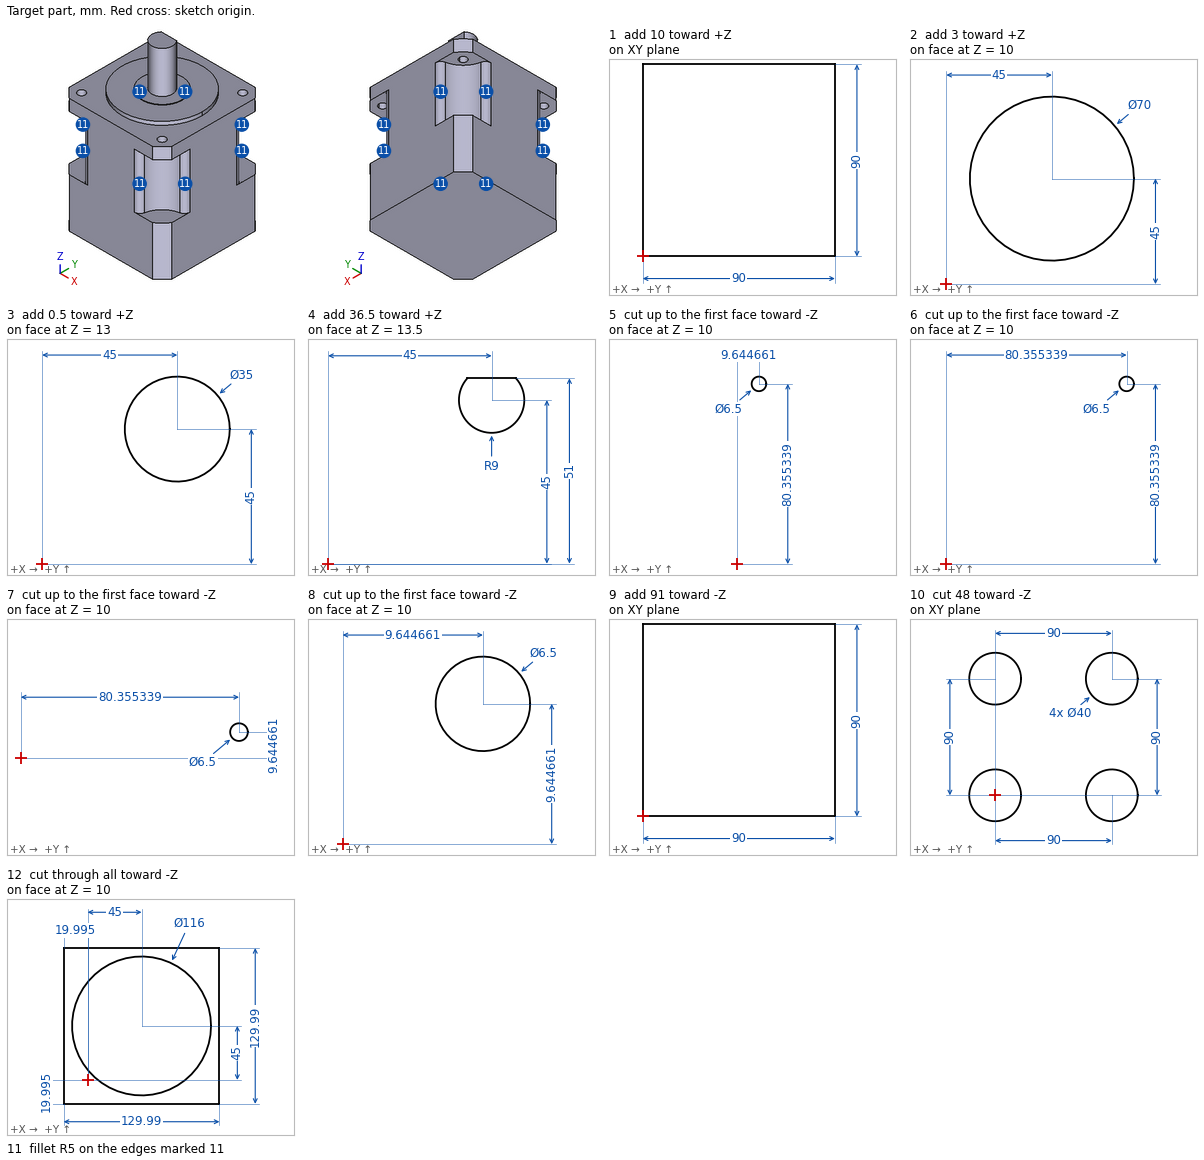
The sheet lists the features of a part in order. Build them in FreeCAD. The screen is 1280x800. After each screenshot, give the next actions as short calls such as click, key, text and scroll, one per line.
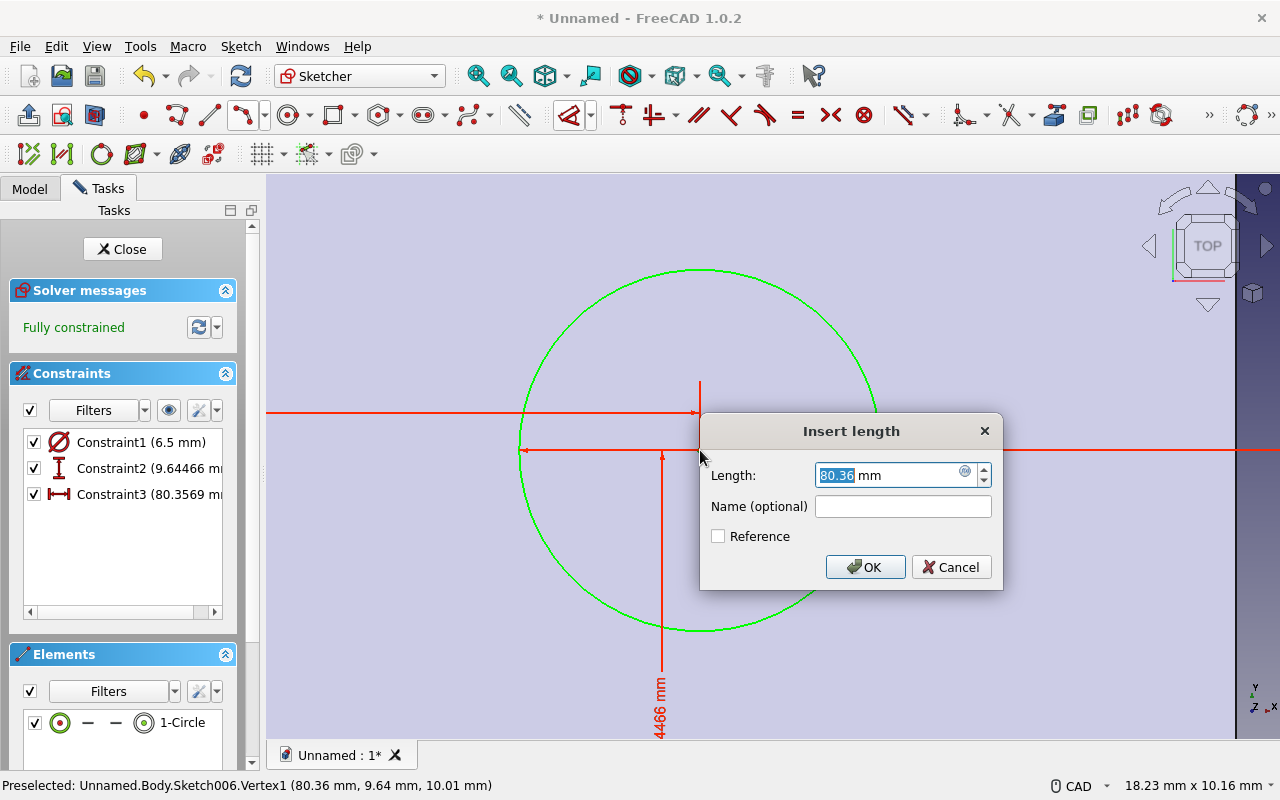
text(80.355339)
key(Return)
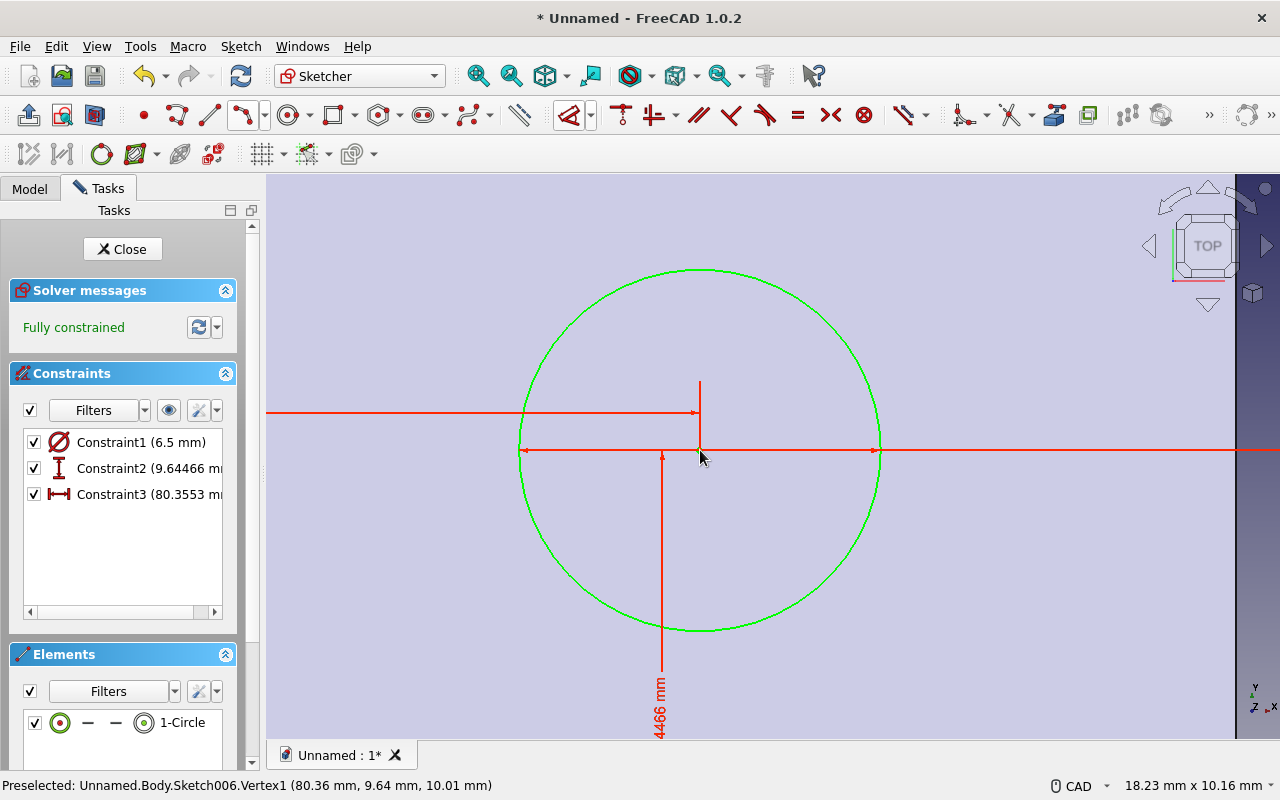
click(123, 249)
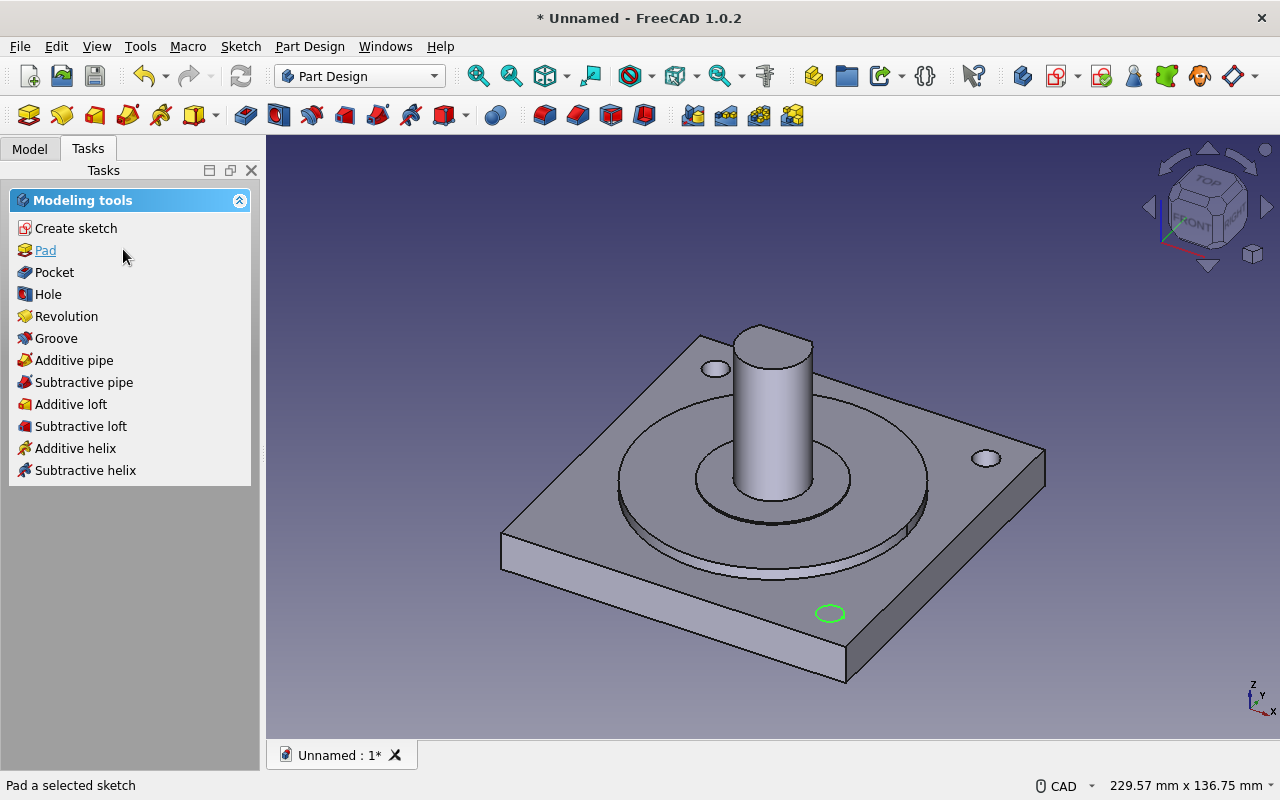
click(246, 116)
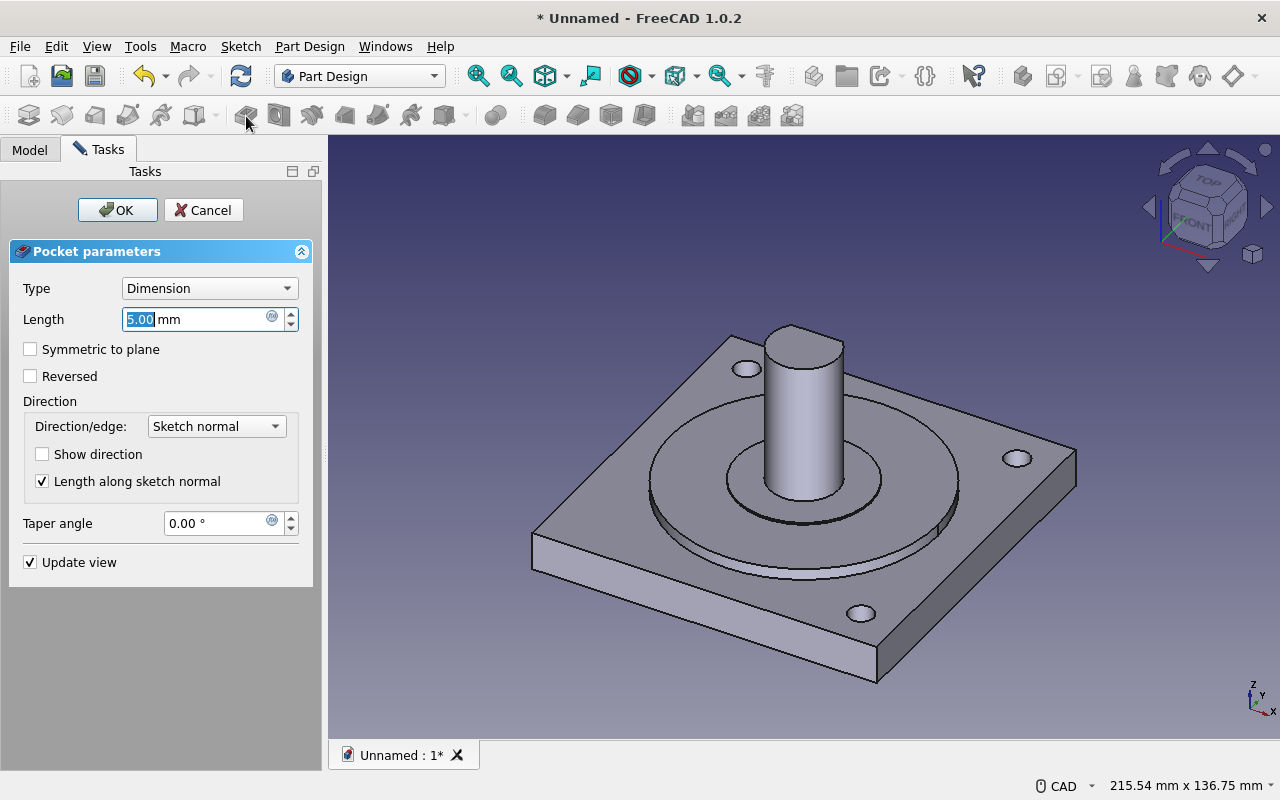
click(210, 288)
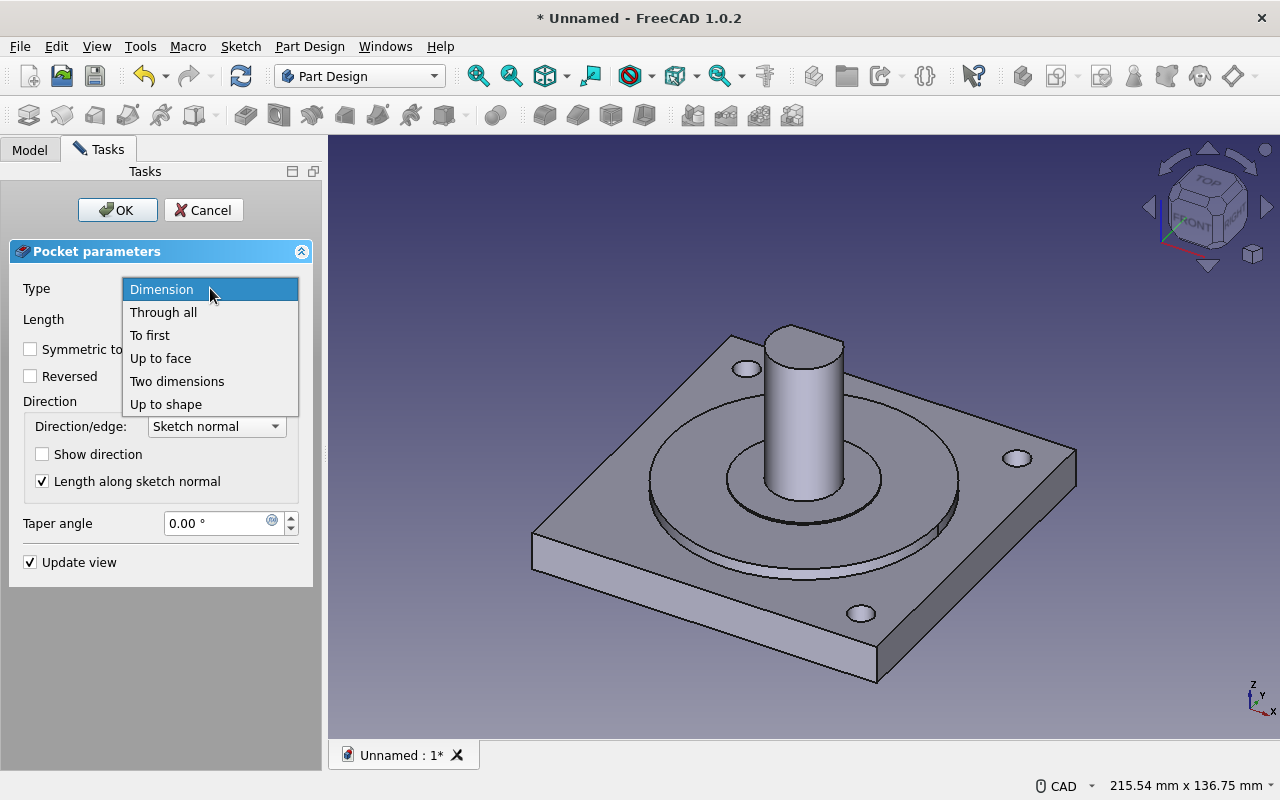
click(208, 336)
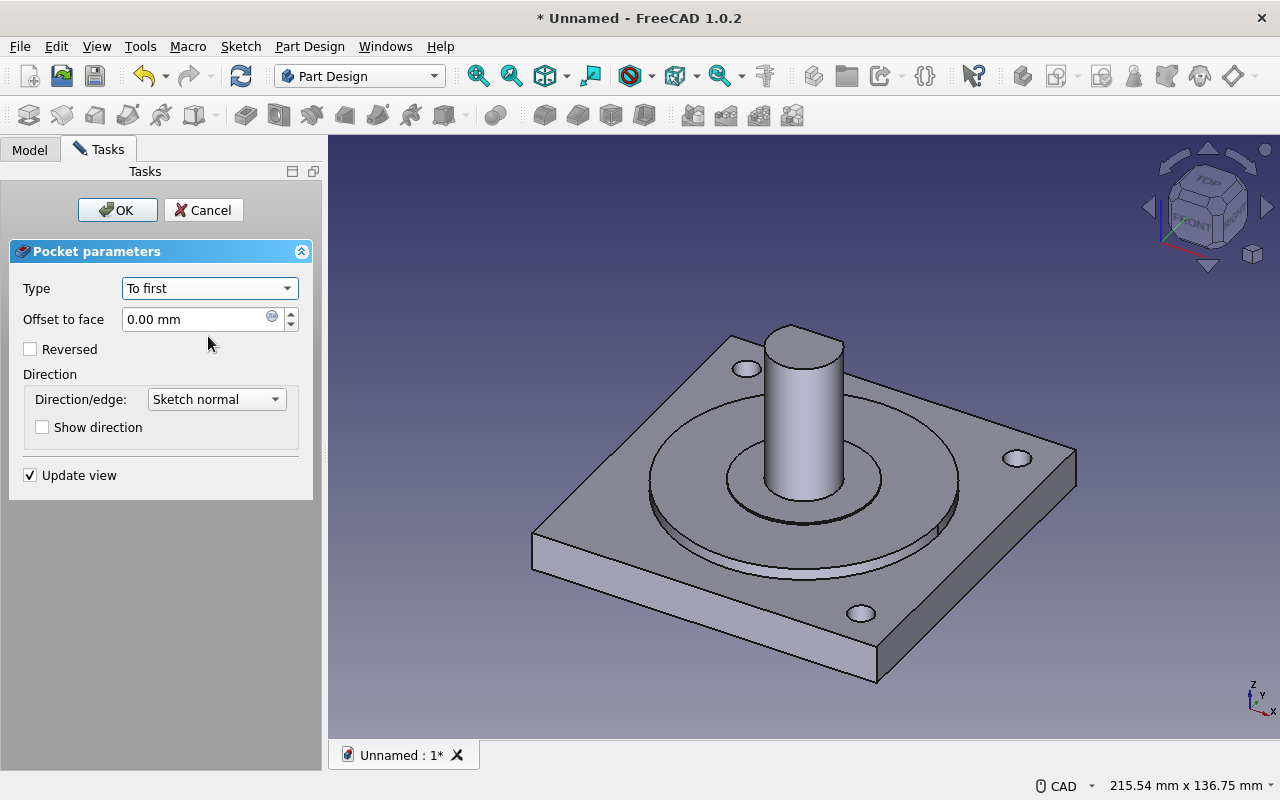
click(118, 210)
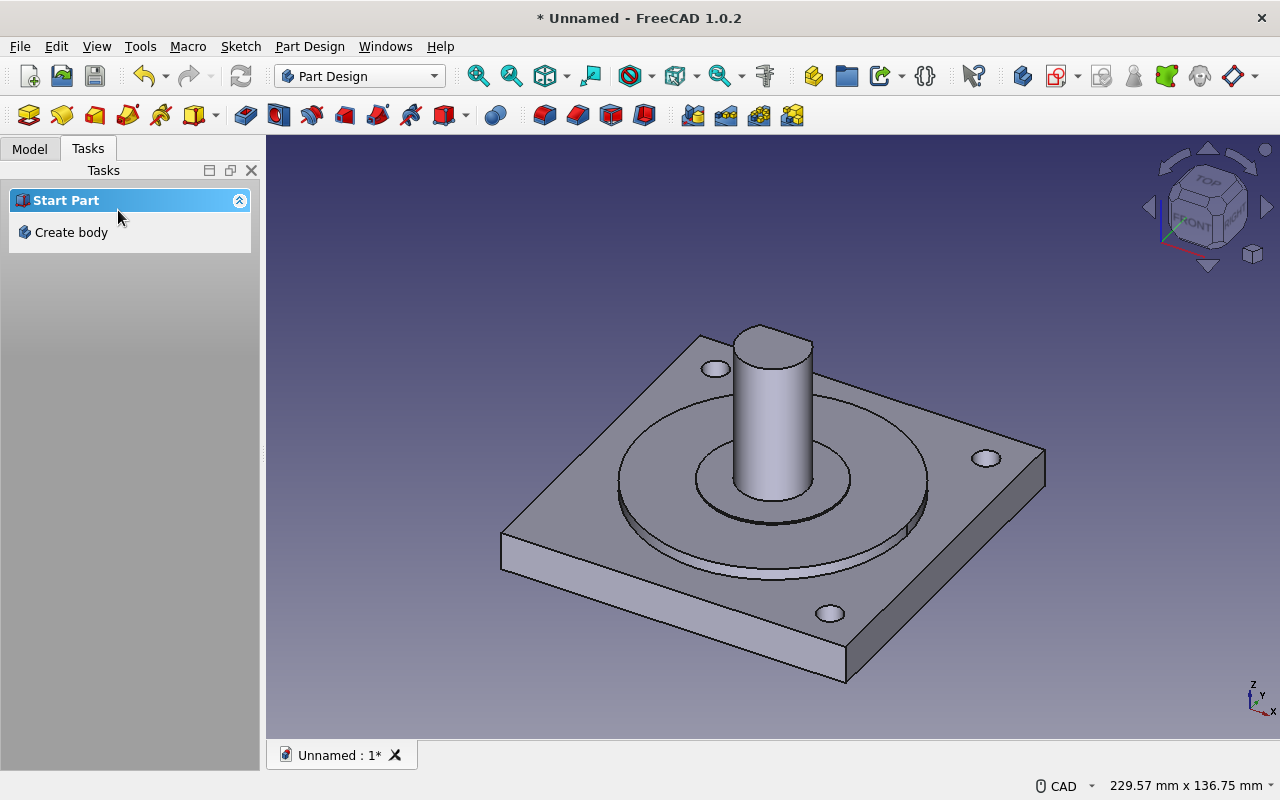
click(977, 483)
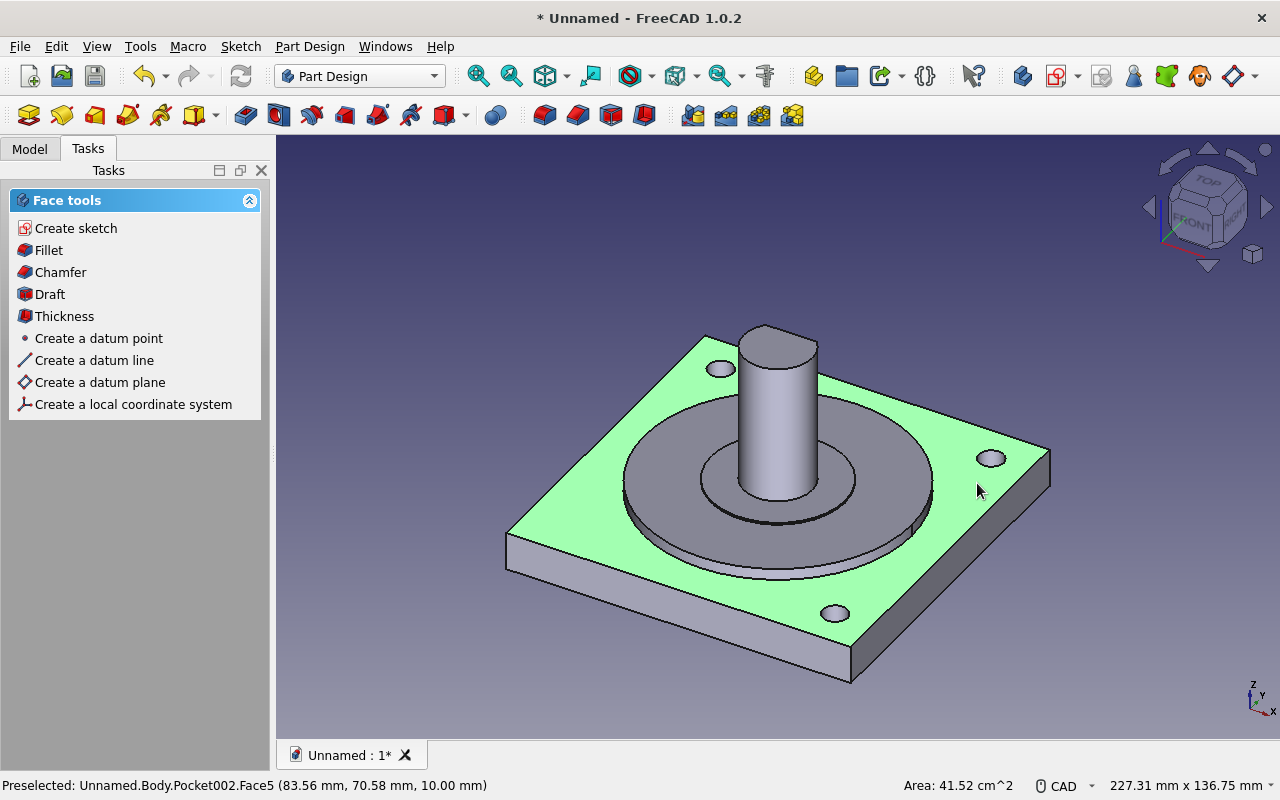
click(1056, 76)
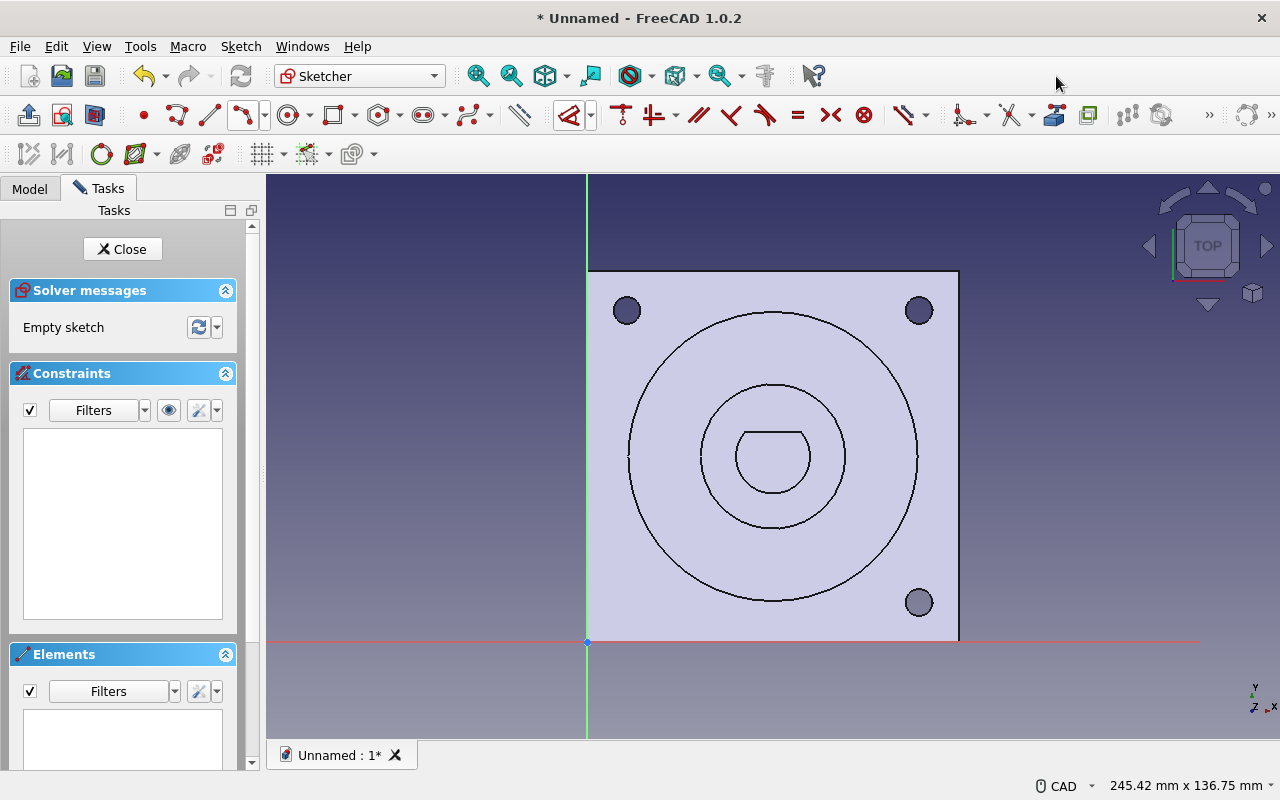
scroll(600, 641, up, 10)